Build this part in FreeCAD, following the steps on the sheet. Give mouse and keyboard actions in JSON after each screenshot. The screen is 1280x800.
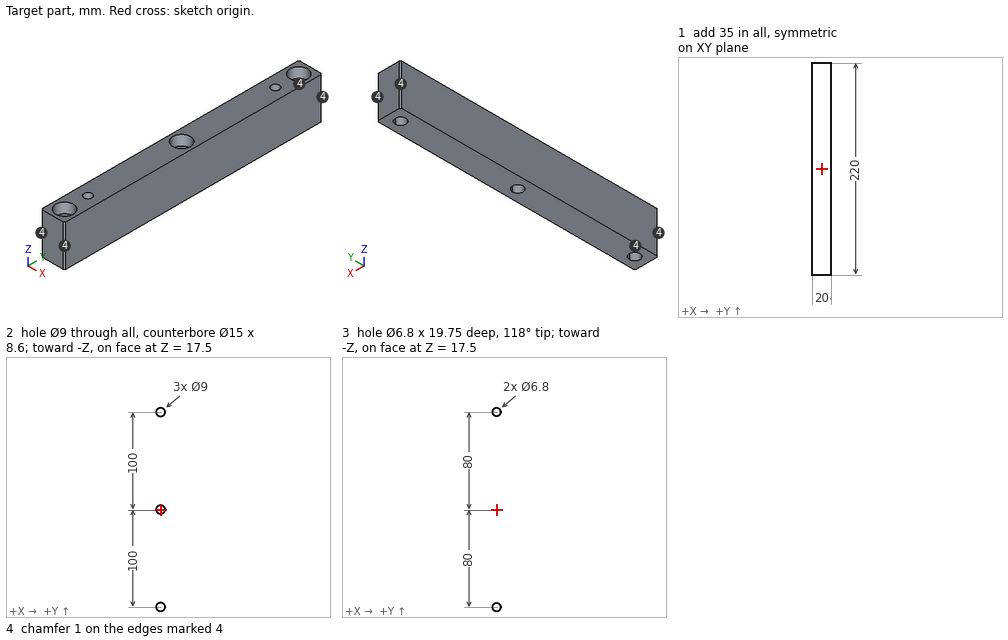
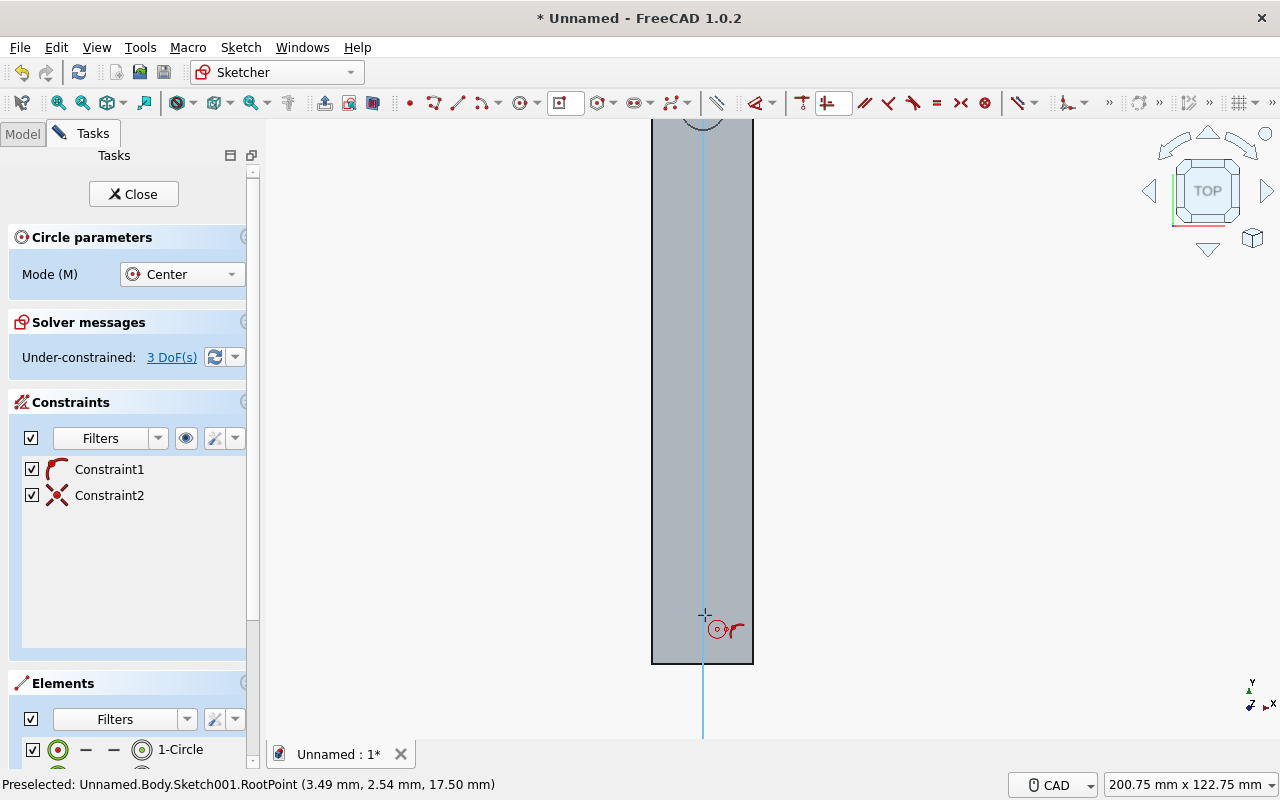
{"action": "left_click", "coordinate": [703, 614]}
{"action": "left_click", "coordinate": [719, 597]}
{"action": "key", "text": "Escape"}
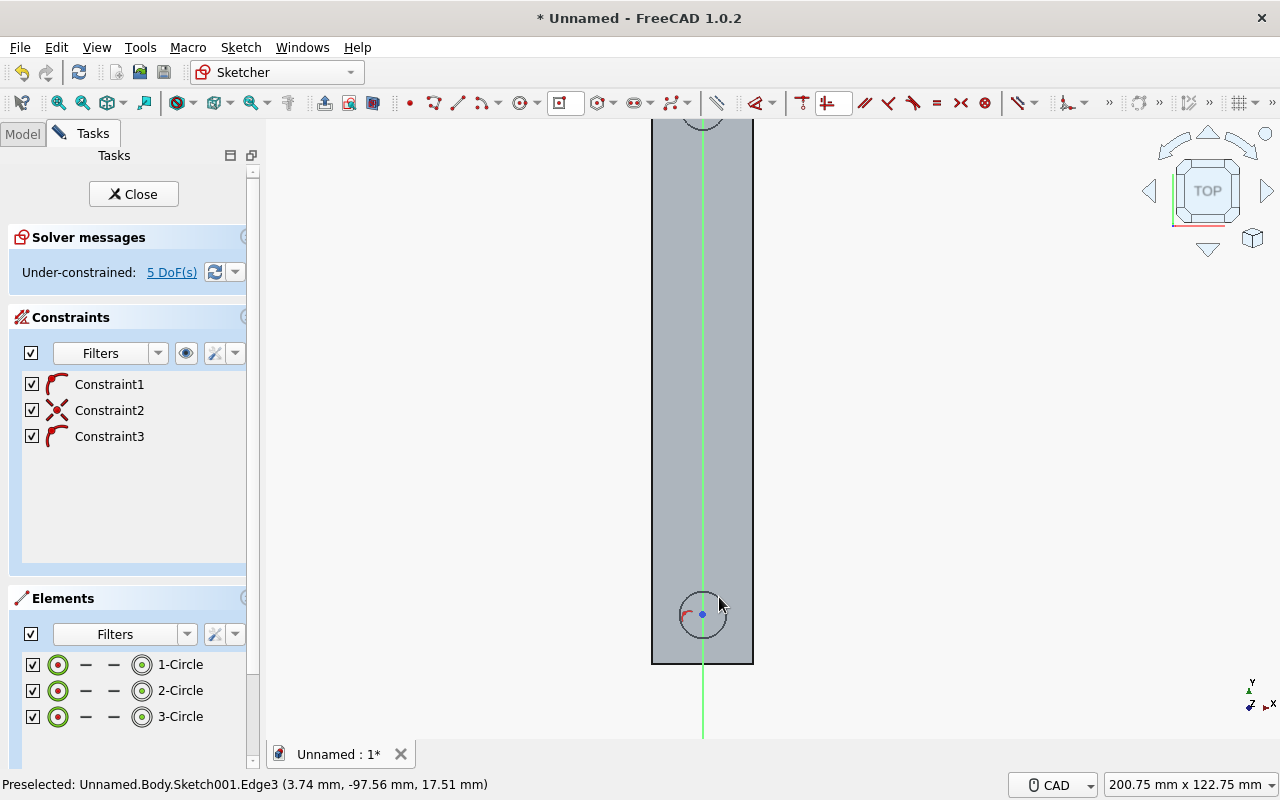
{"action": "scroll", "coordinate": [705, 616], "scroll_direction": "down", "scroll_amount": 5}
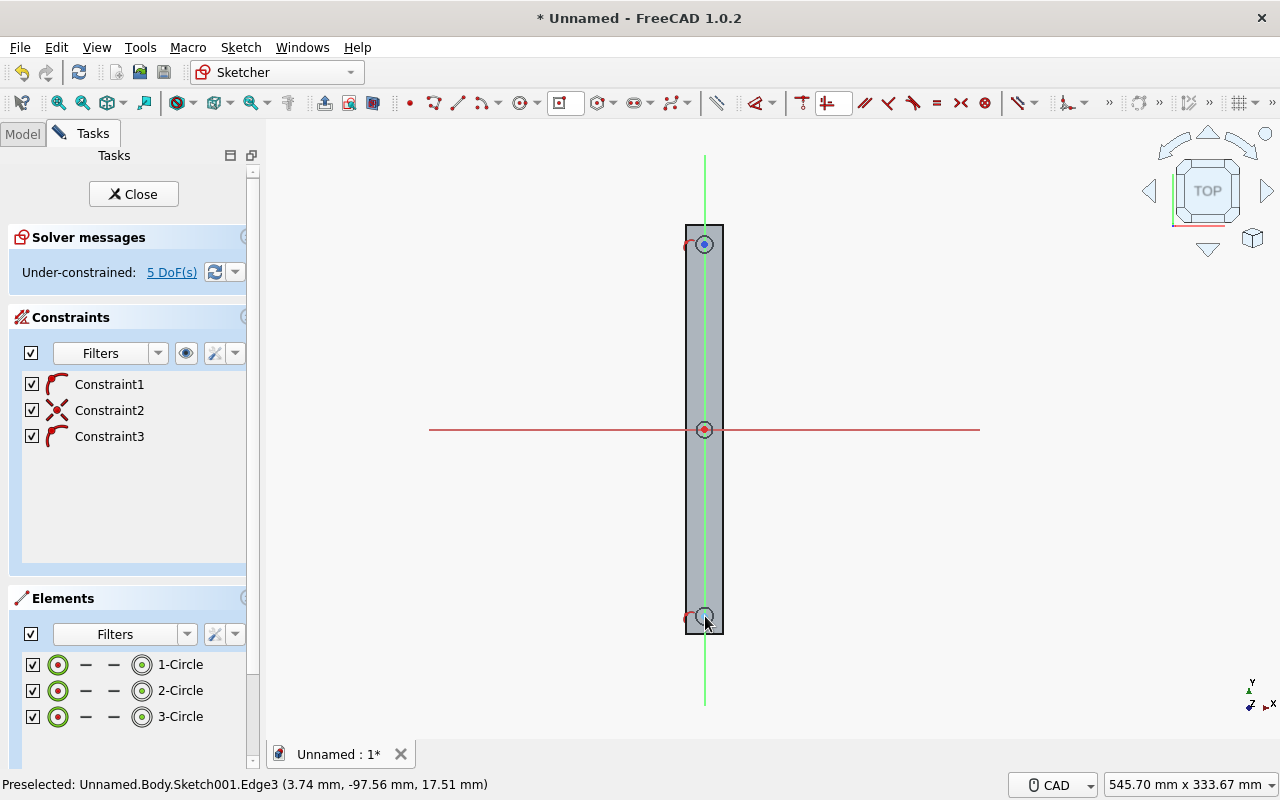
{"action": "scroll", "coordinate": [710, 239], "scroll_direction": "up", "scroll_amount": 5}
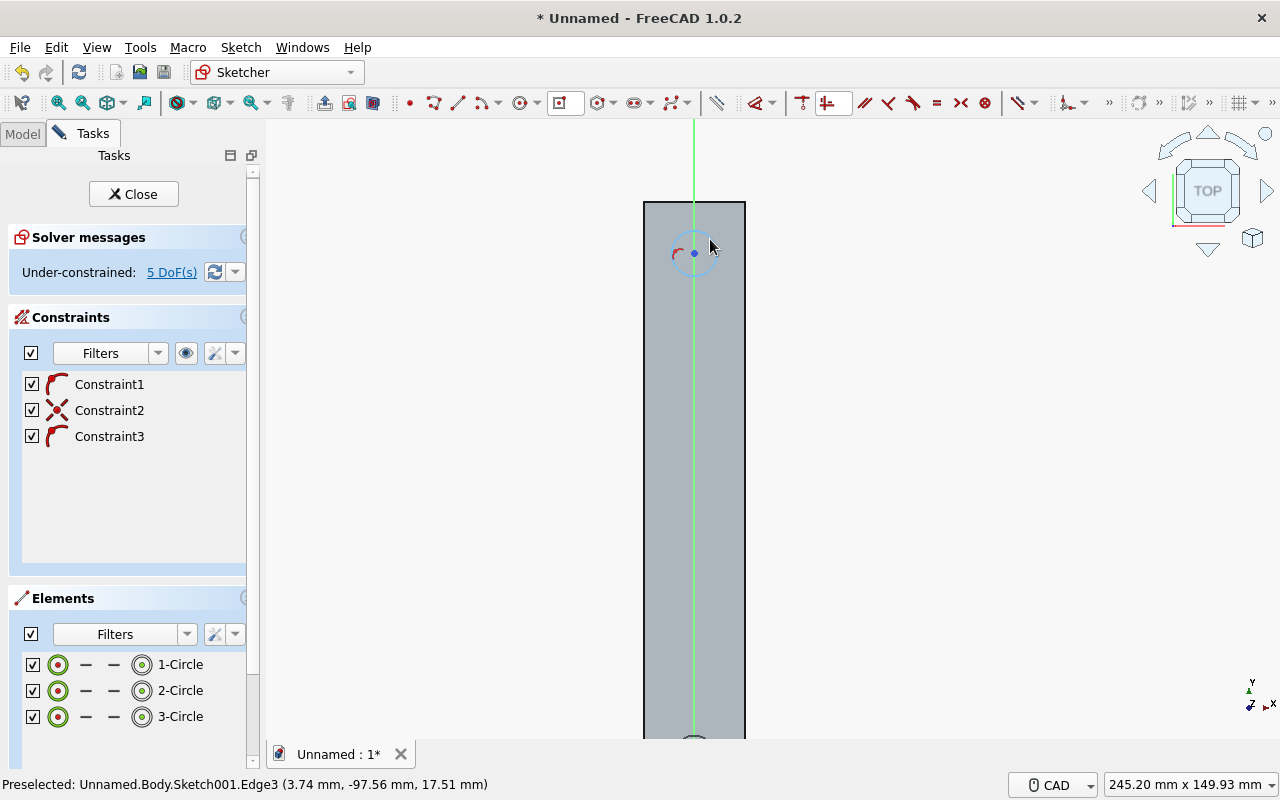
{"action": "left_click", "coordinate": [710, 238]}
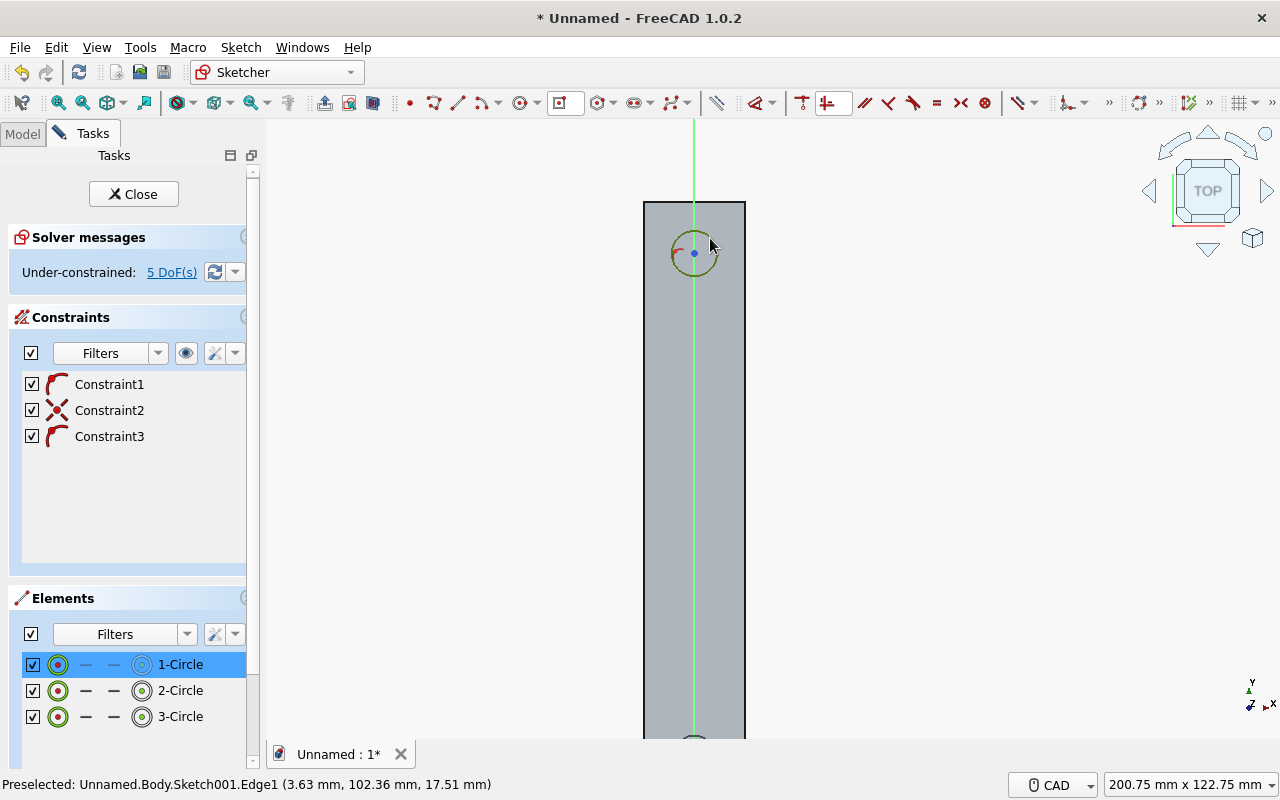
{"action": "scroll", "coordinate": [710, 238], "scroll_direction": "down", "scroll_amount": 5}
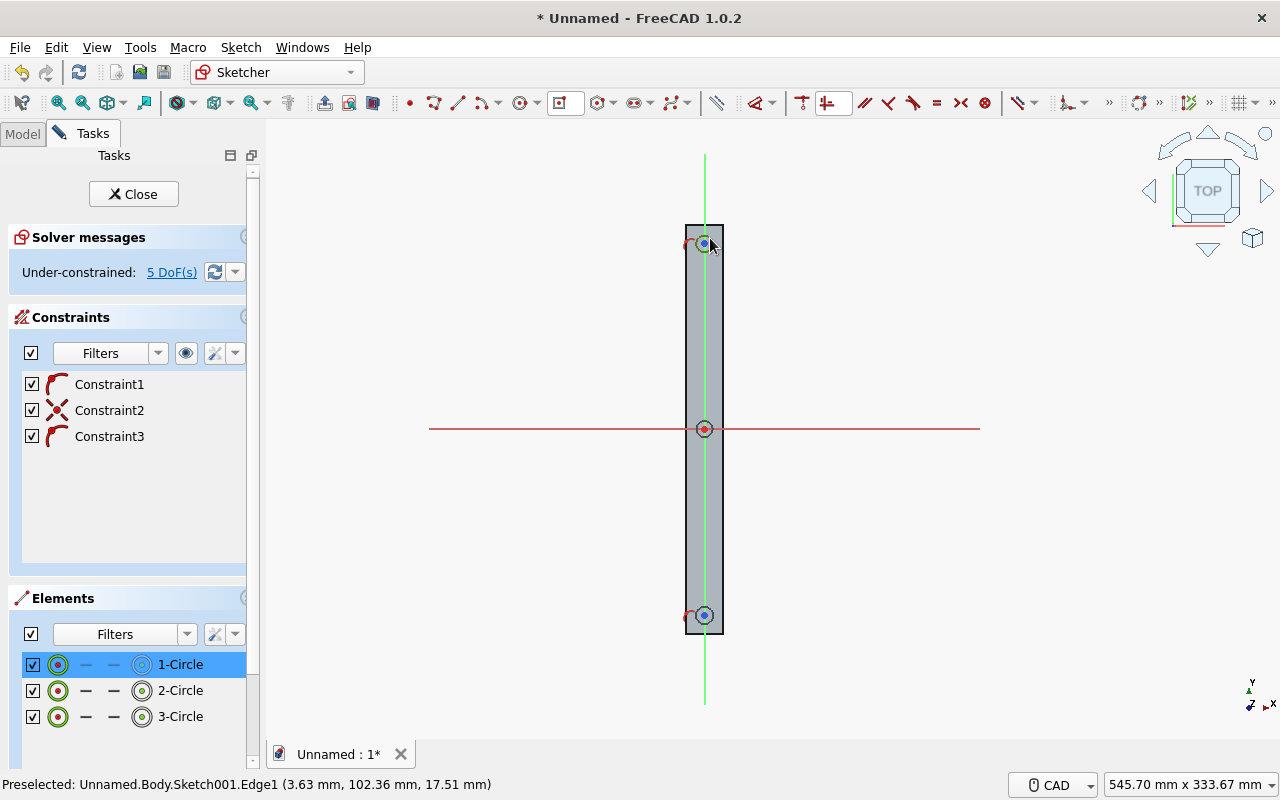
{"action": "scroll", "coordinate": [710, 424], "scroll_direction": "up", "scroll_amount": 5}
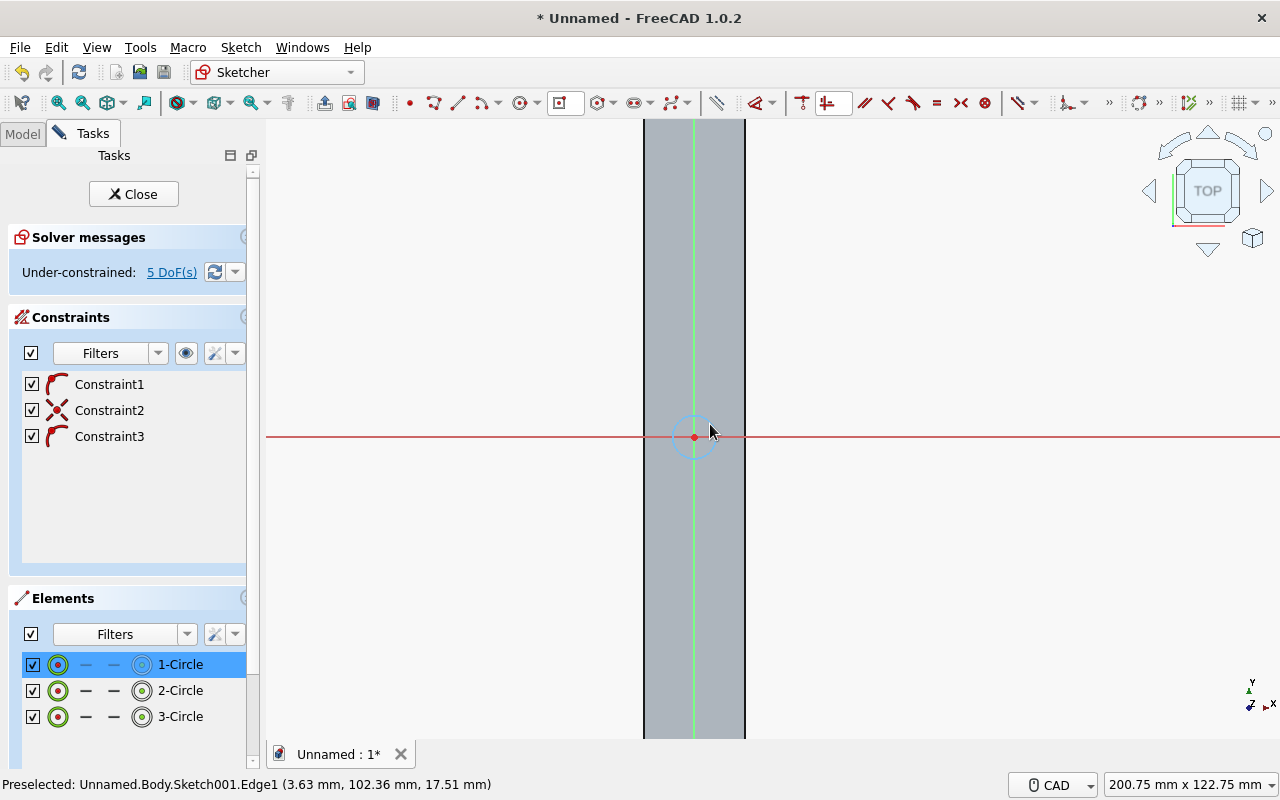
{"action": "left_click", "coordinate": [710, 422]}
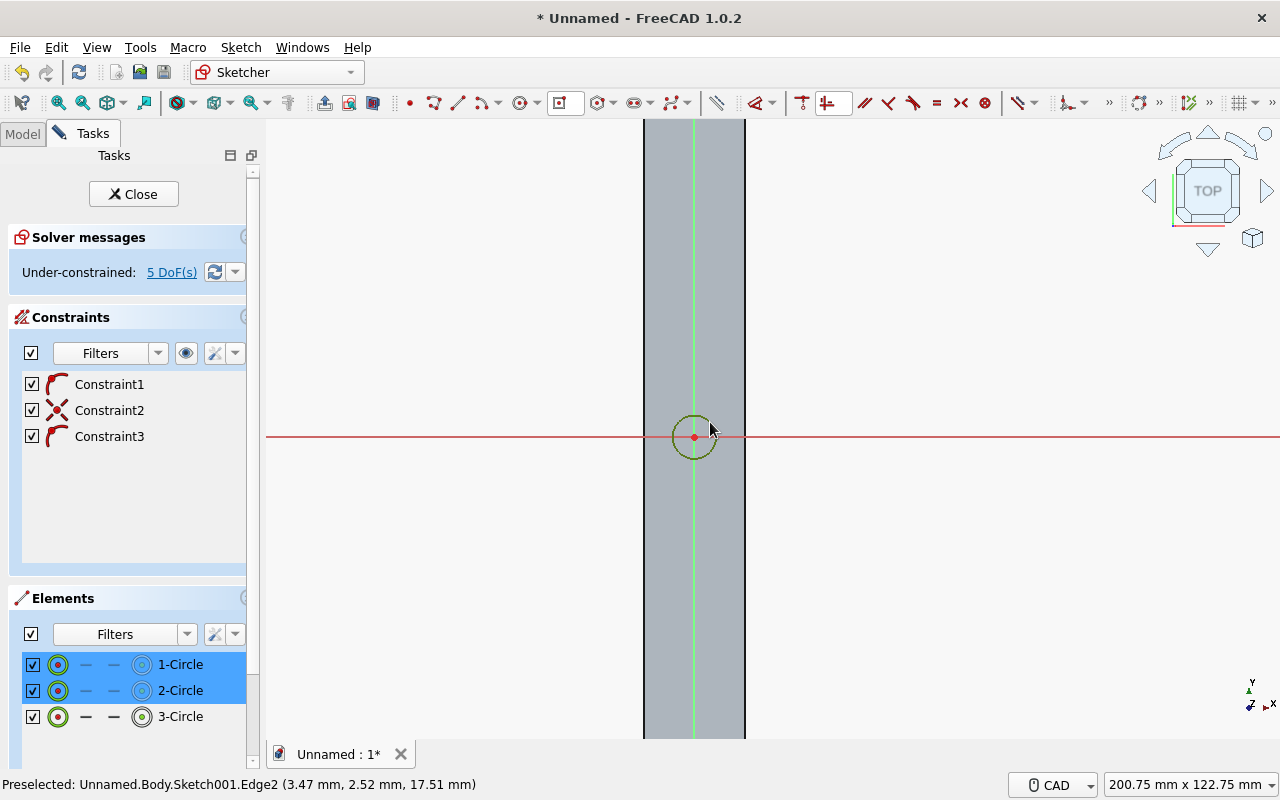
{"action": "scroll", "coordinate": [710, 424], "scroll_direction": "down", "scroll_amount": 5}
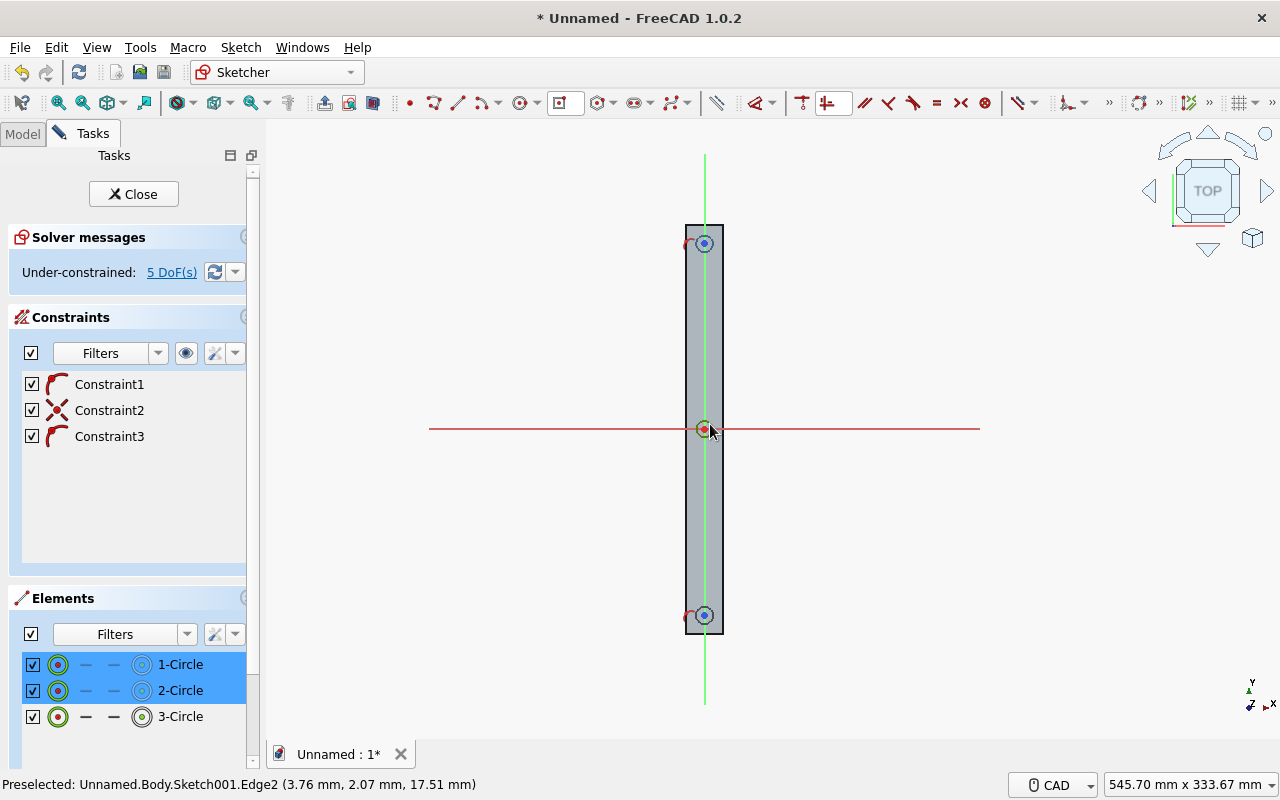
{"action": "scroll", "coordinate": [711, 609], "scroll_direction": "up", "scroll_amount": 5}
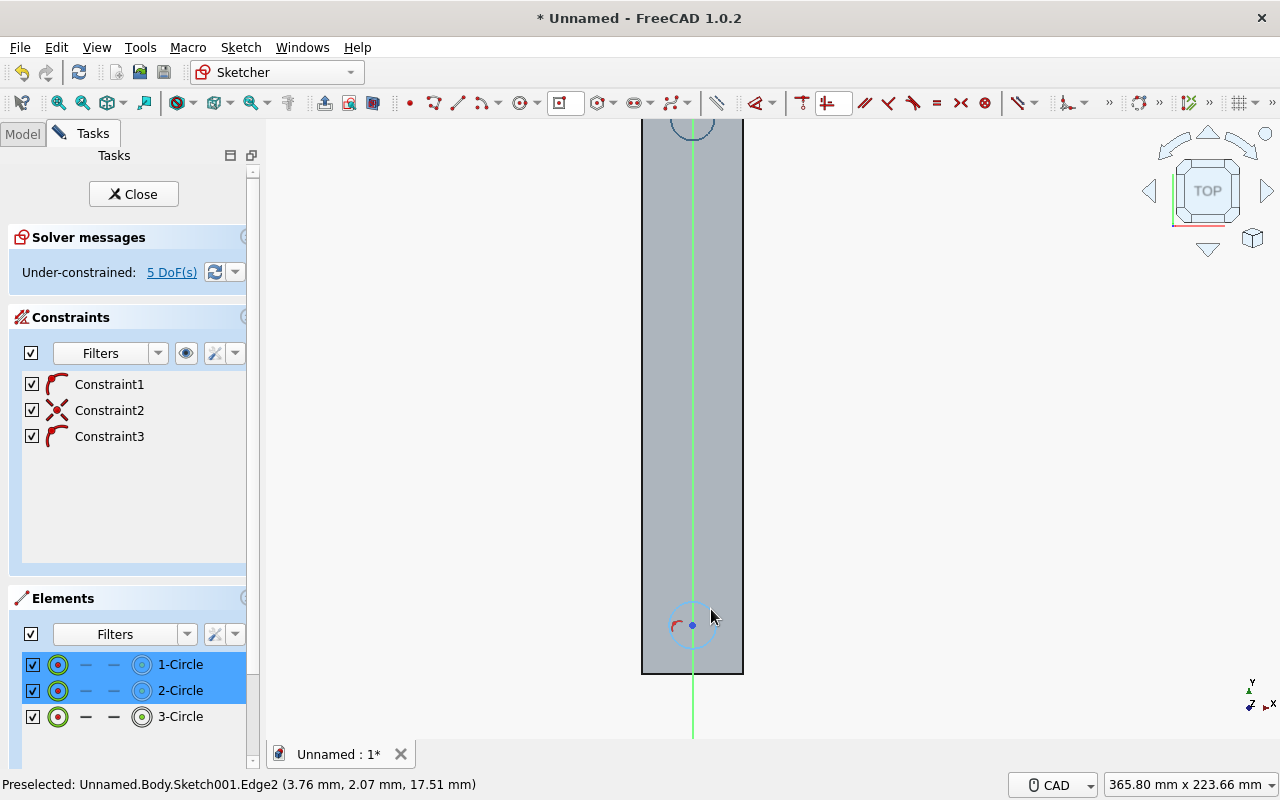
{"action": "left_click", "coordinate": [709, 609]}